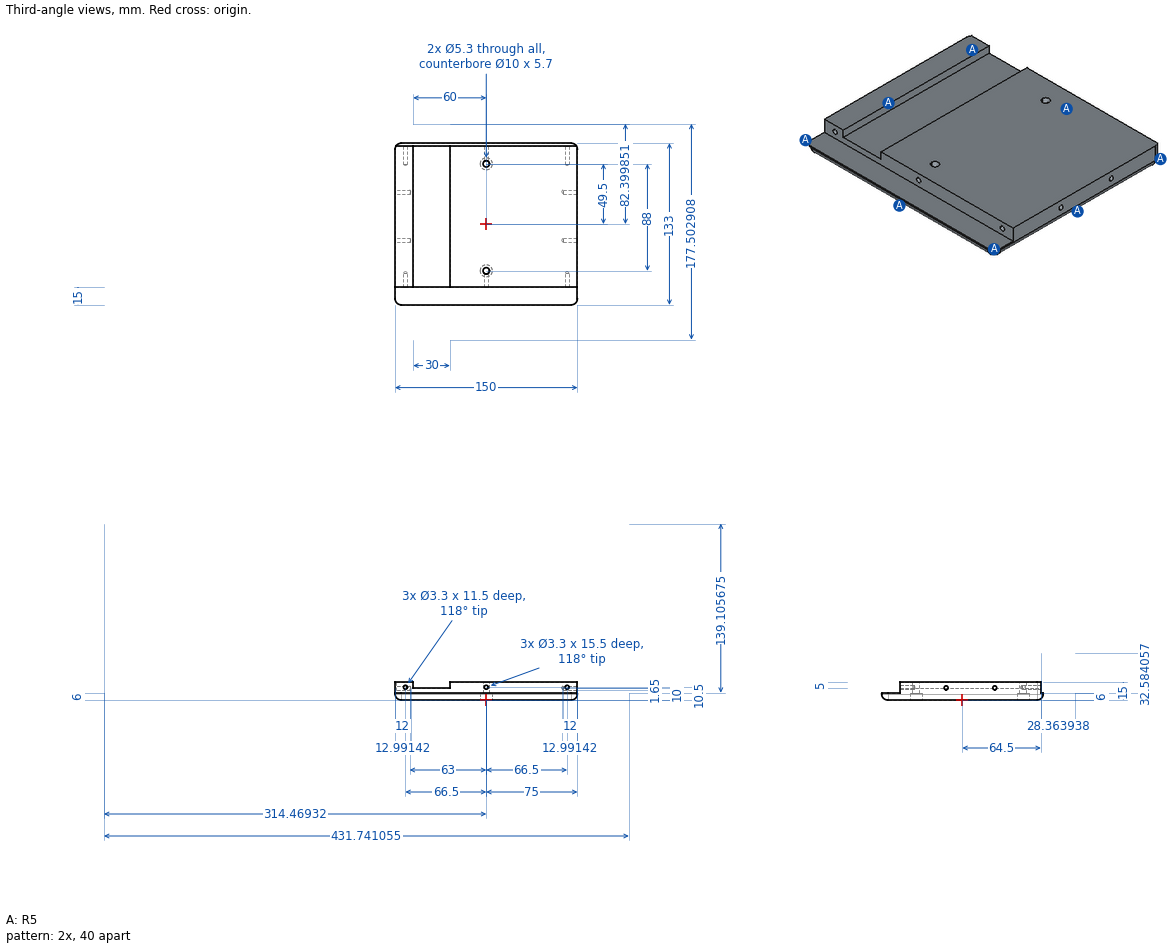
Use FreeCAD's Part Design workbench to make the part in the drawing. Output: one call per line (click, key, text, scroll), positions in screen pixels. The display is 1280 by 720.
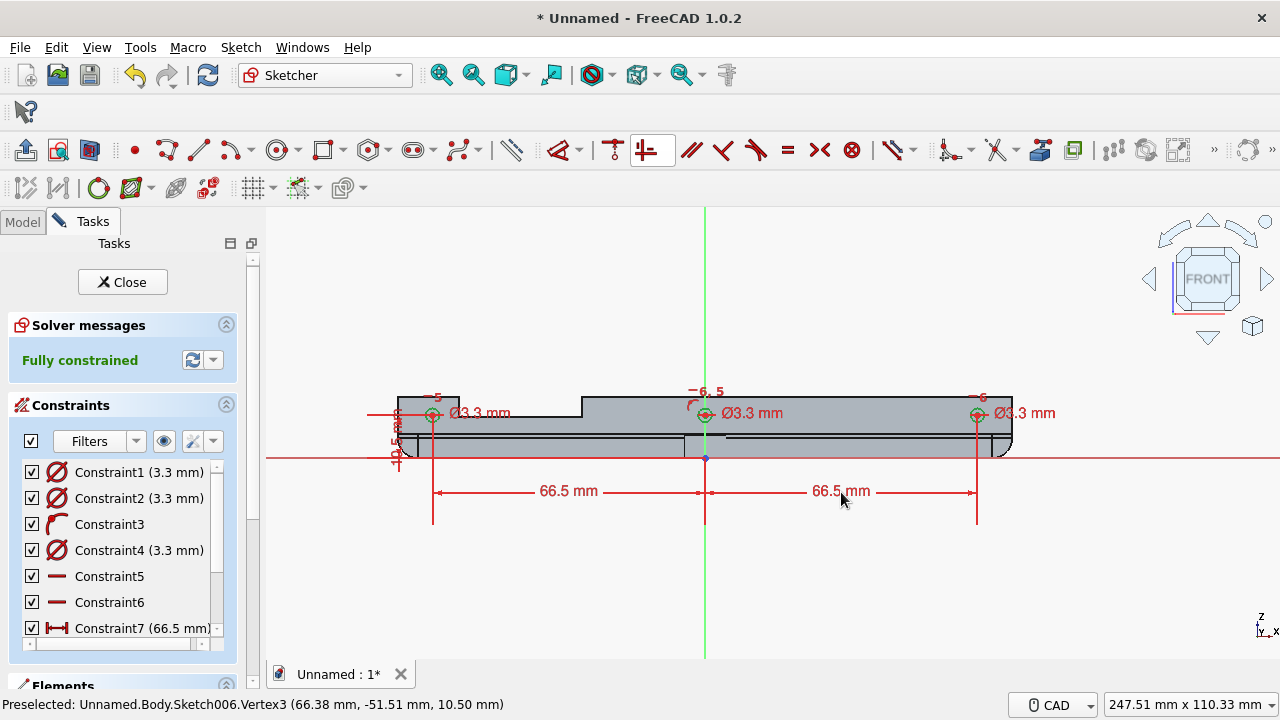
click(123, 282)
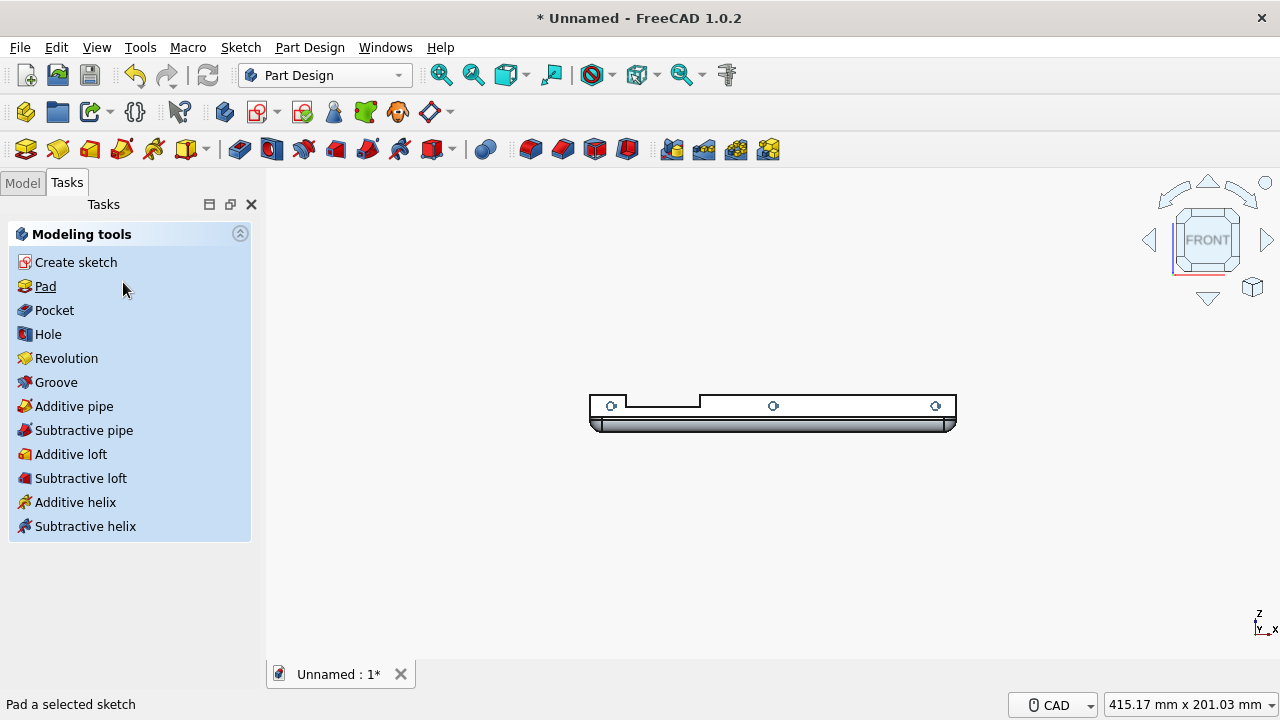
click(272, 150)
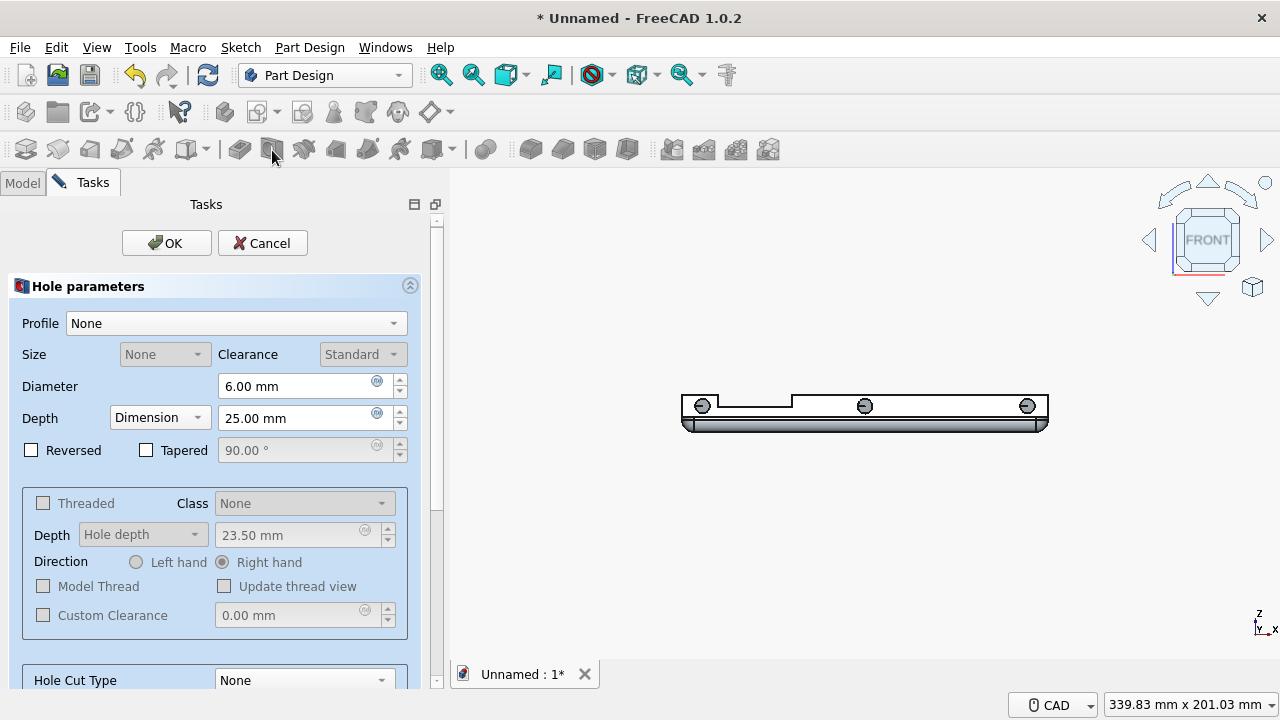
triple_click(305, 386)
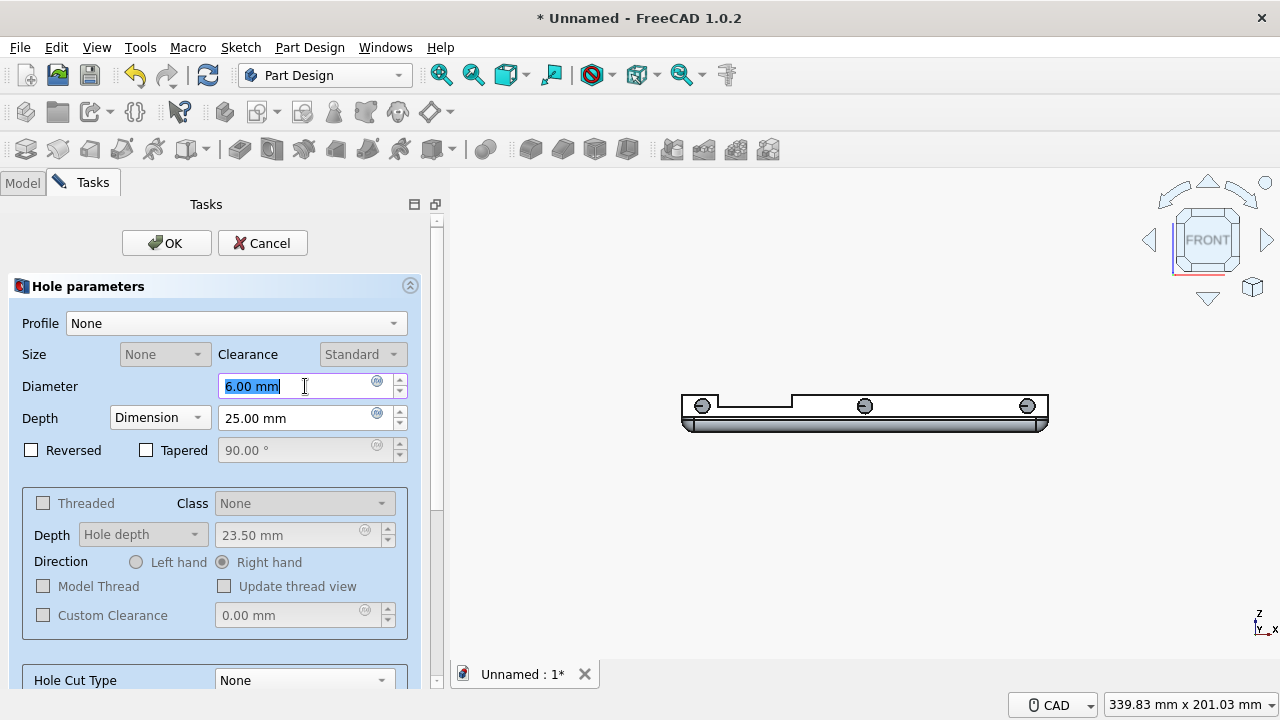
text(3.3)
key(Tab)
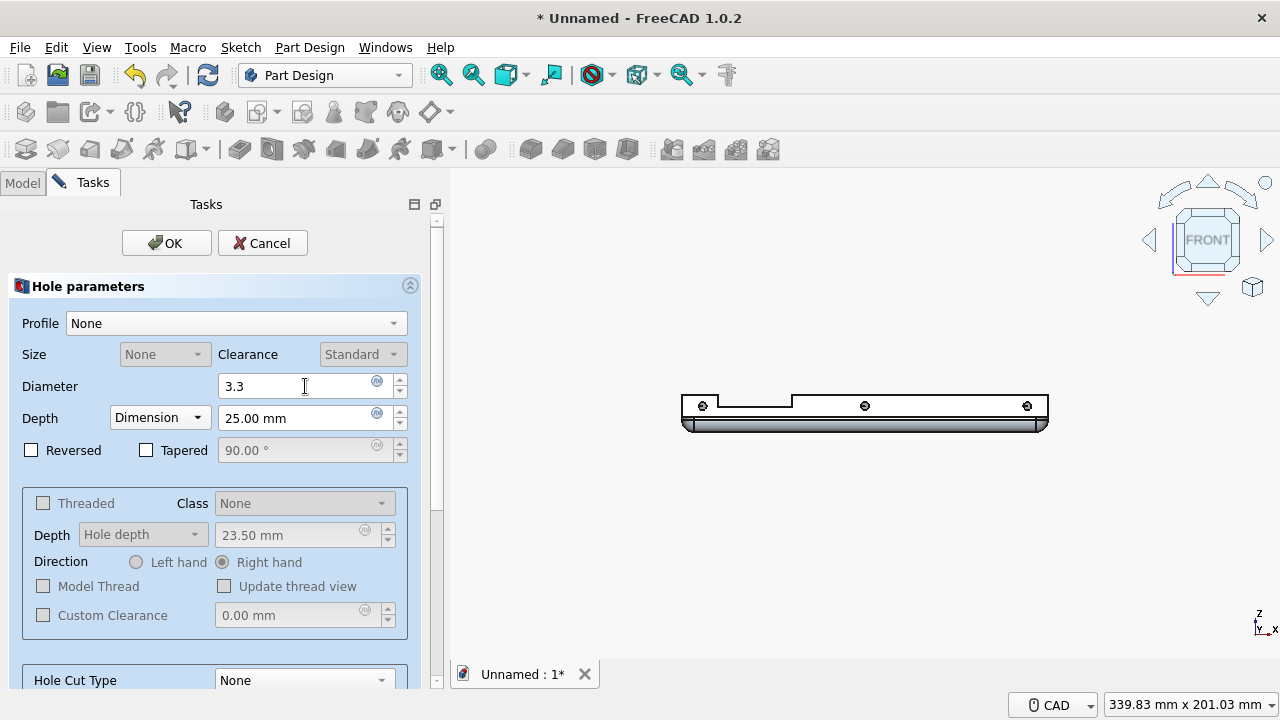
triple_click(305, 418)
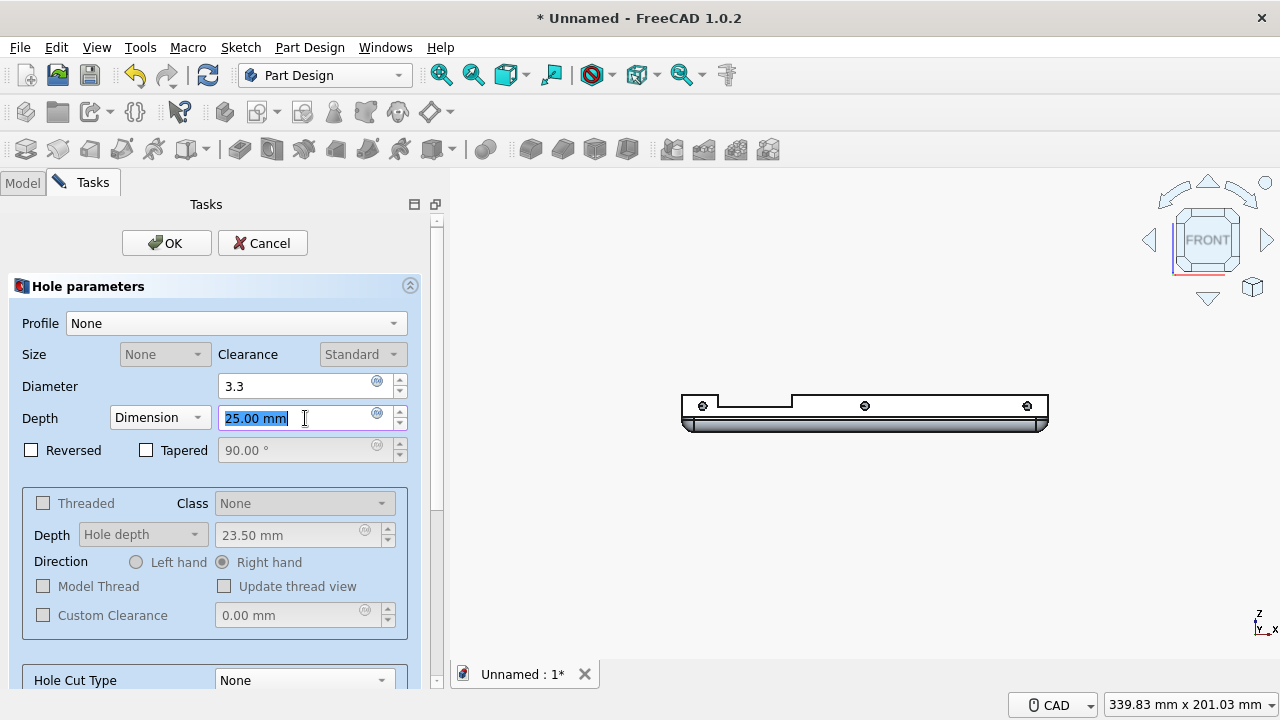
text(11.5)
key(Tab)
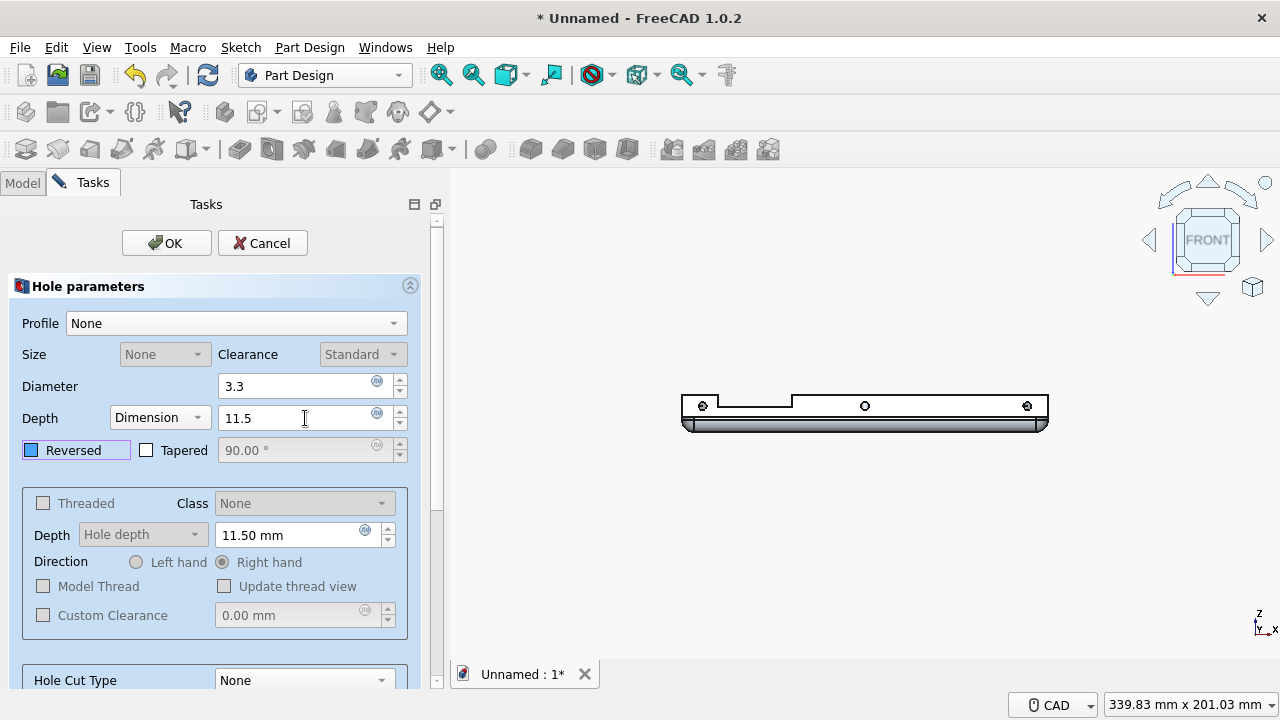
click(167, 243)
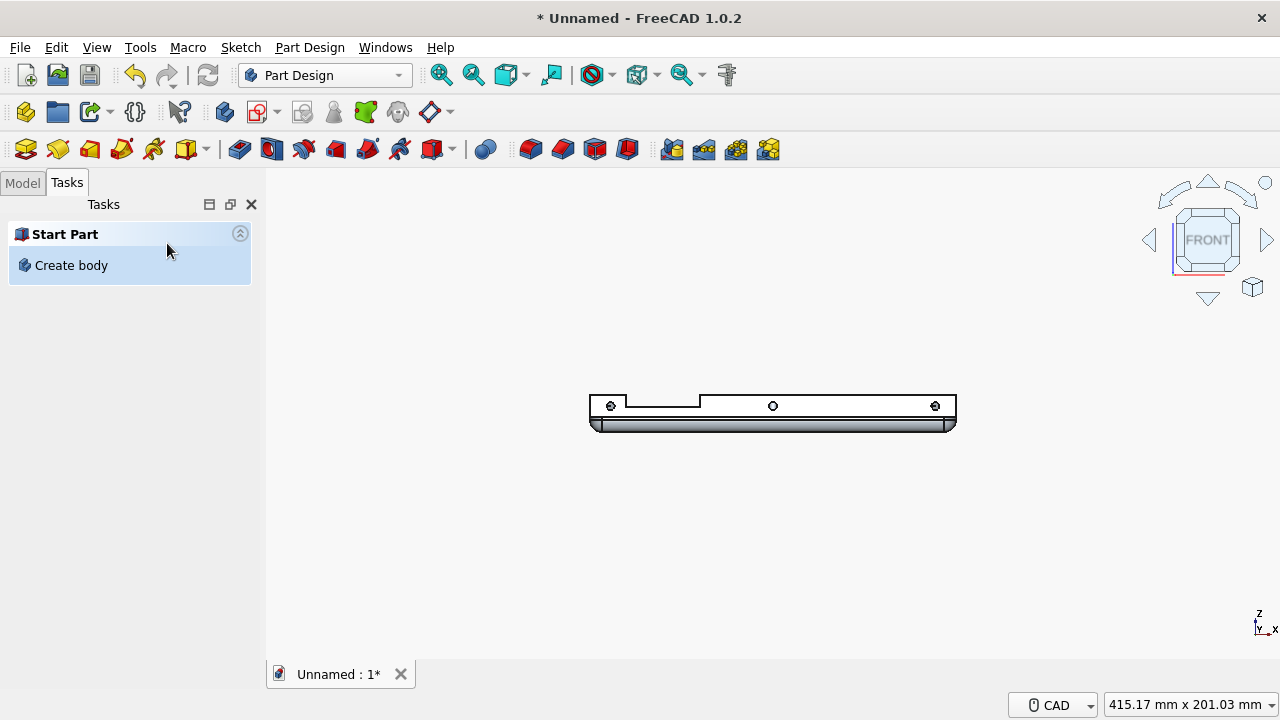
click(442, 76)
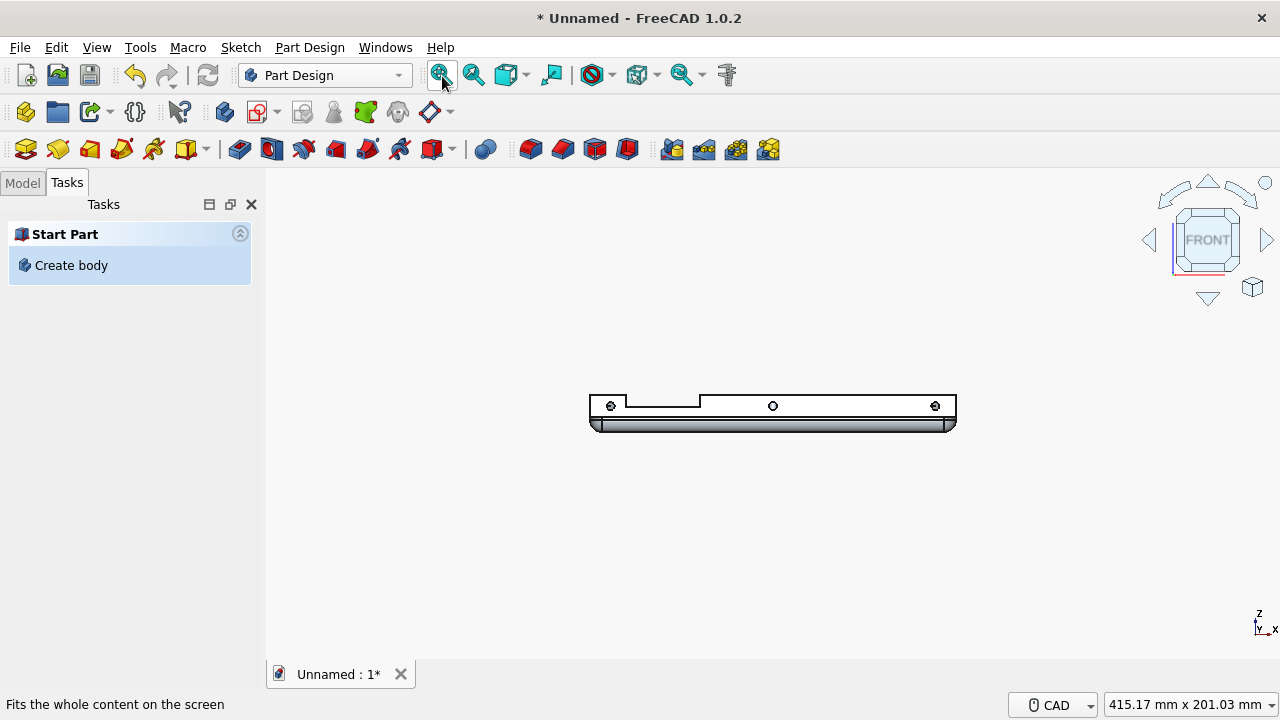
click(23, 182)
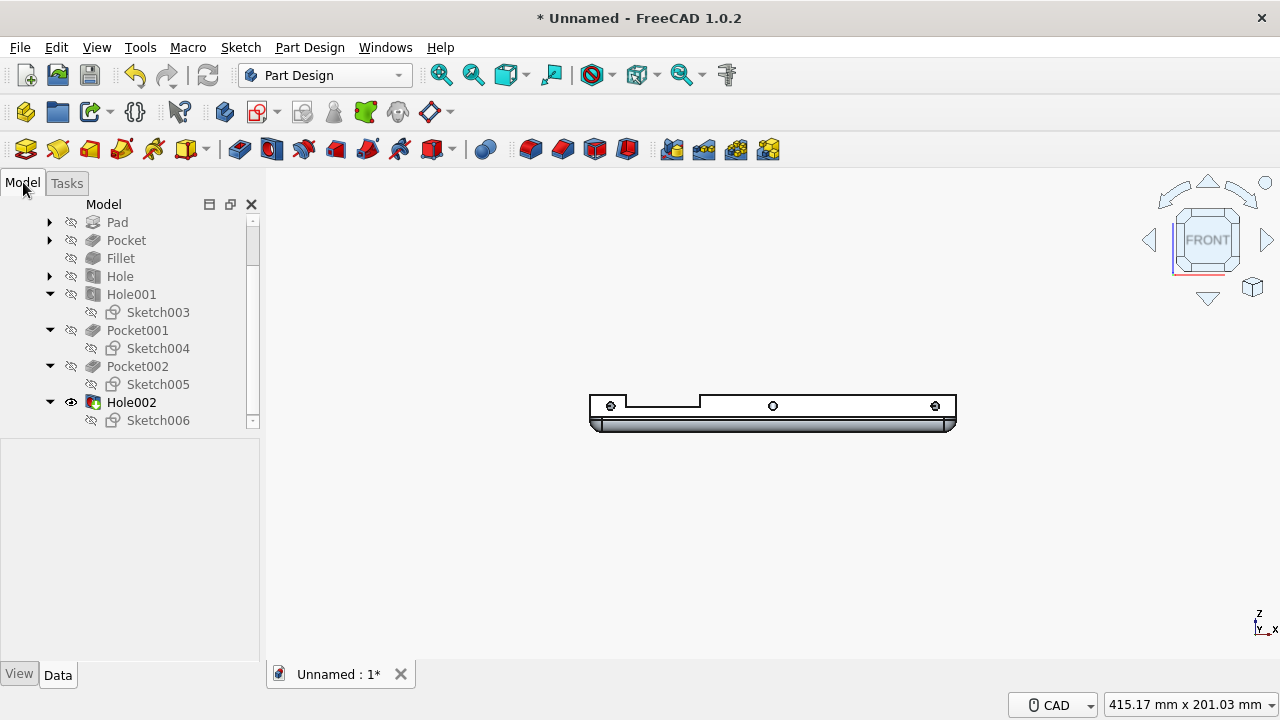
scroll(140, 326, down, 3)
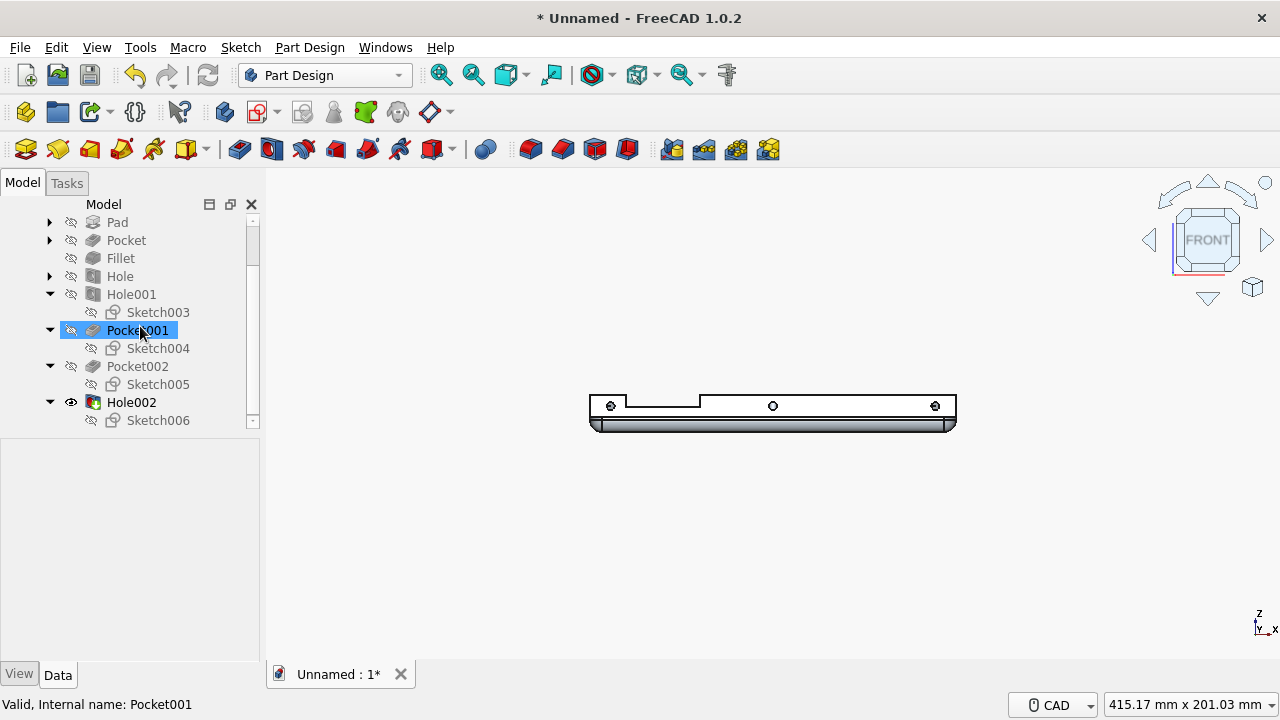
scroll(140, 326, up, 15)